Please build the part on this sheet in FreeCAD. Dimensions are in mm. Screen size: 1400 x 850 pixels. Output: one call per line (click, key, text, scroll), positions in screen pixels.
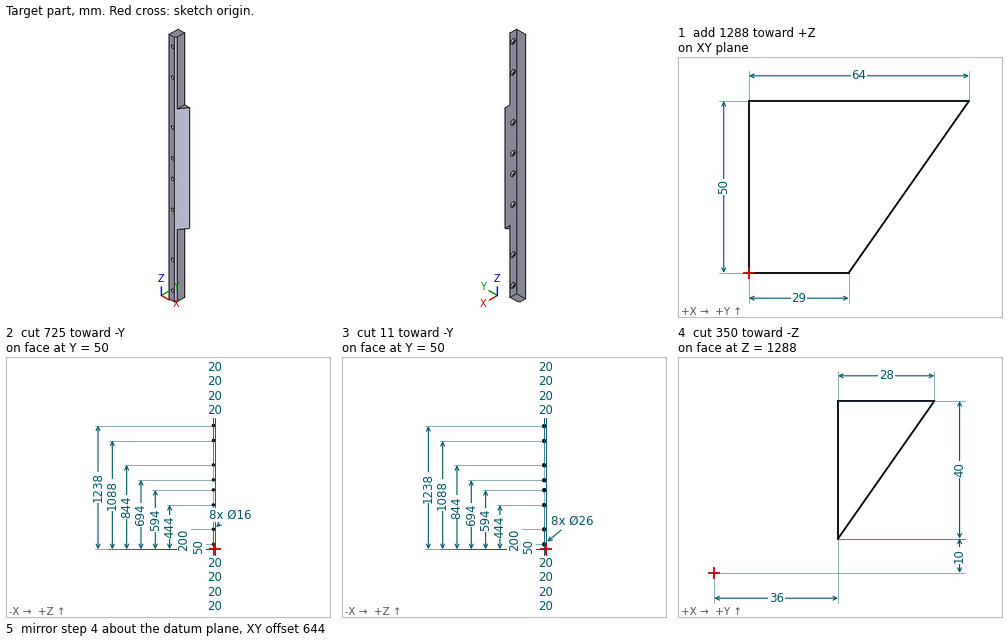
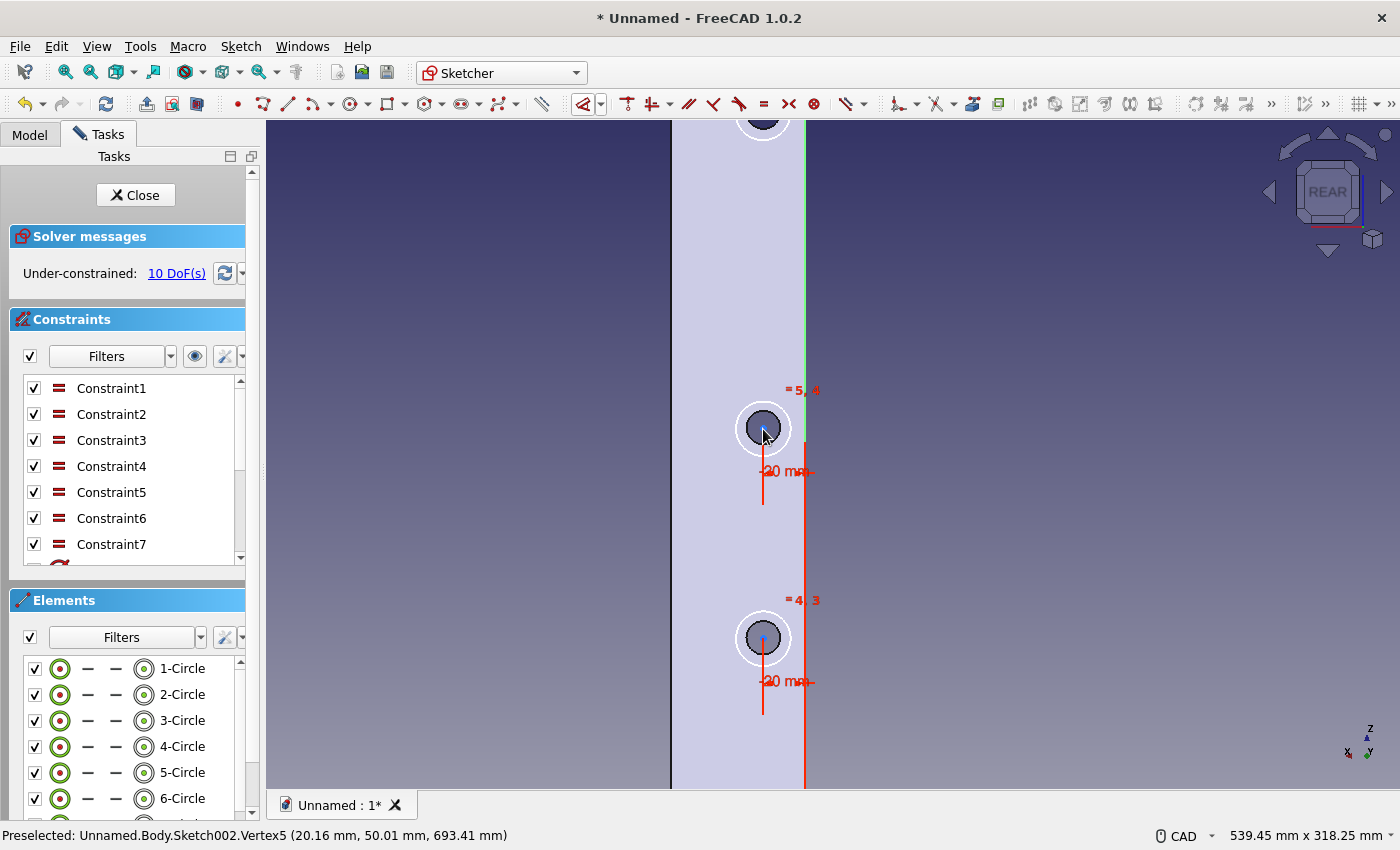
scroll(763, 431, down, 9)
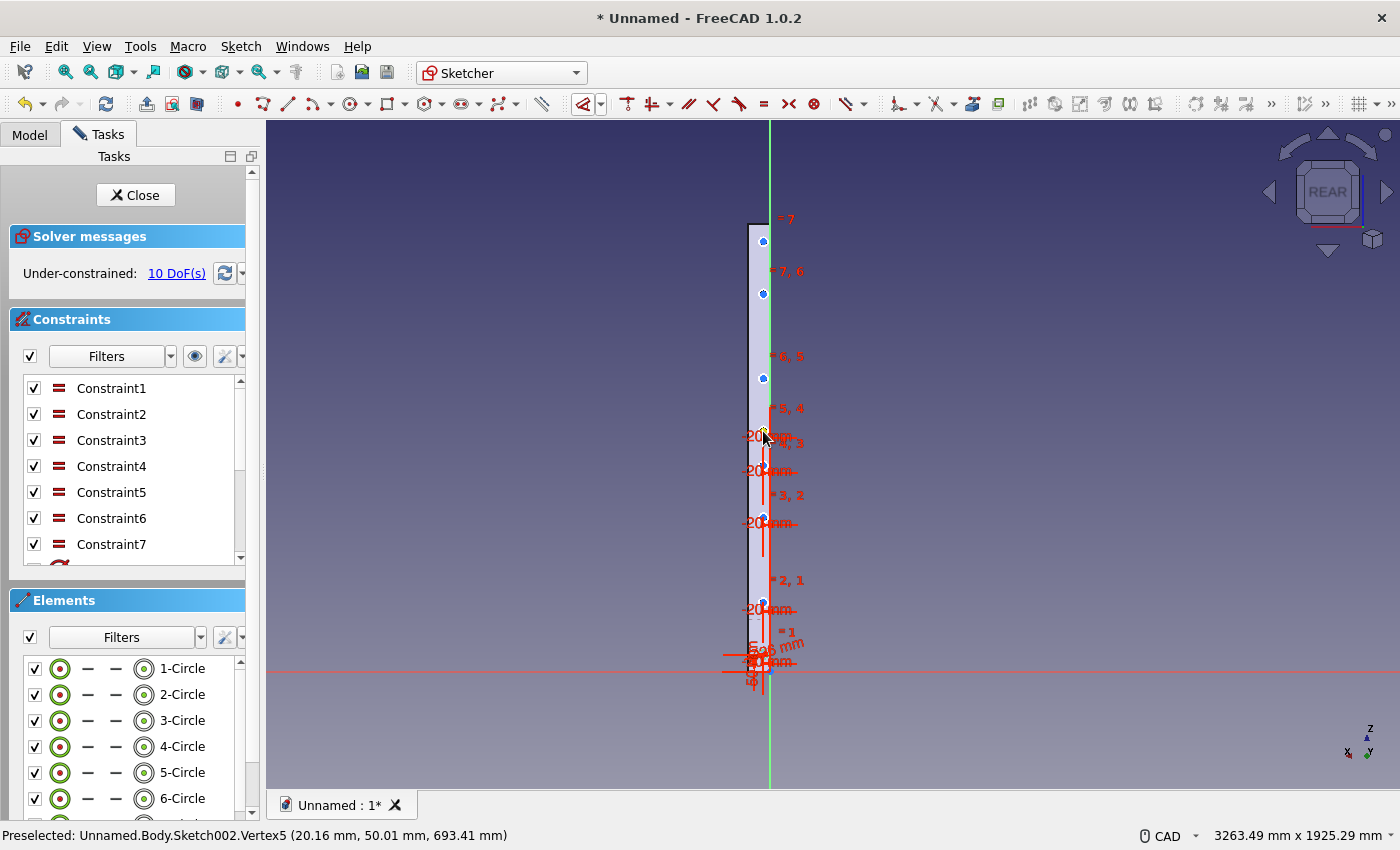
scroll(763, 379, up, 9)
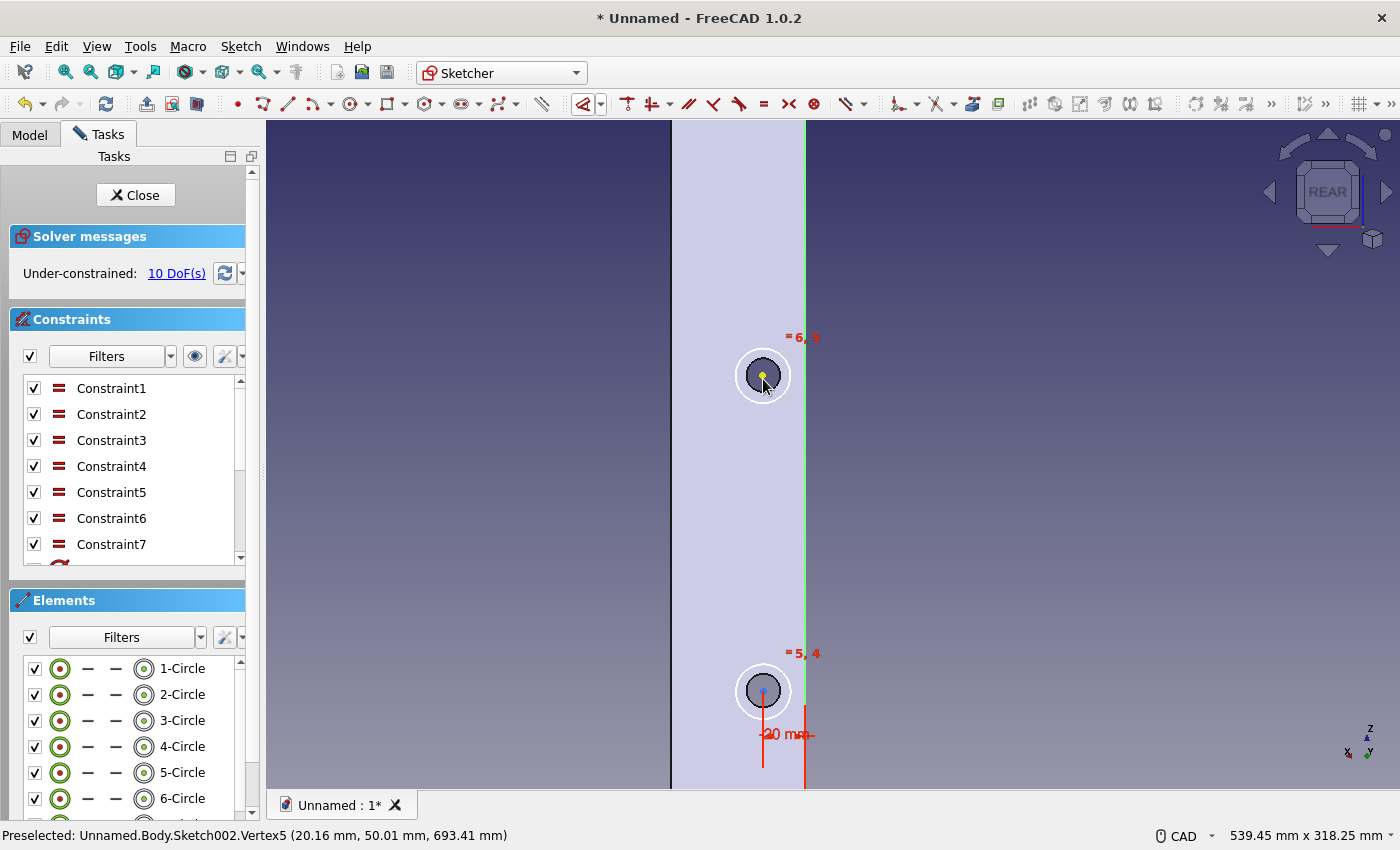
click(763, 376)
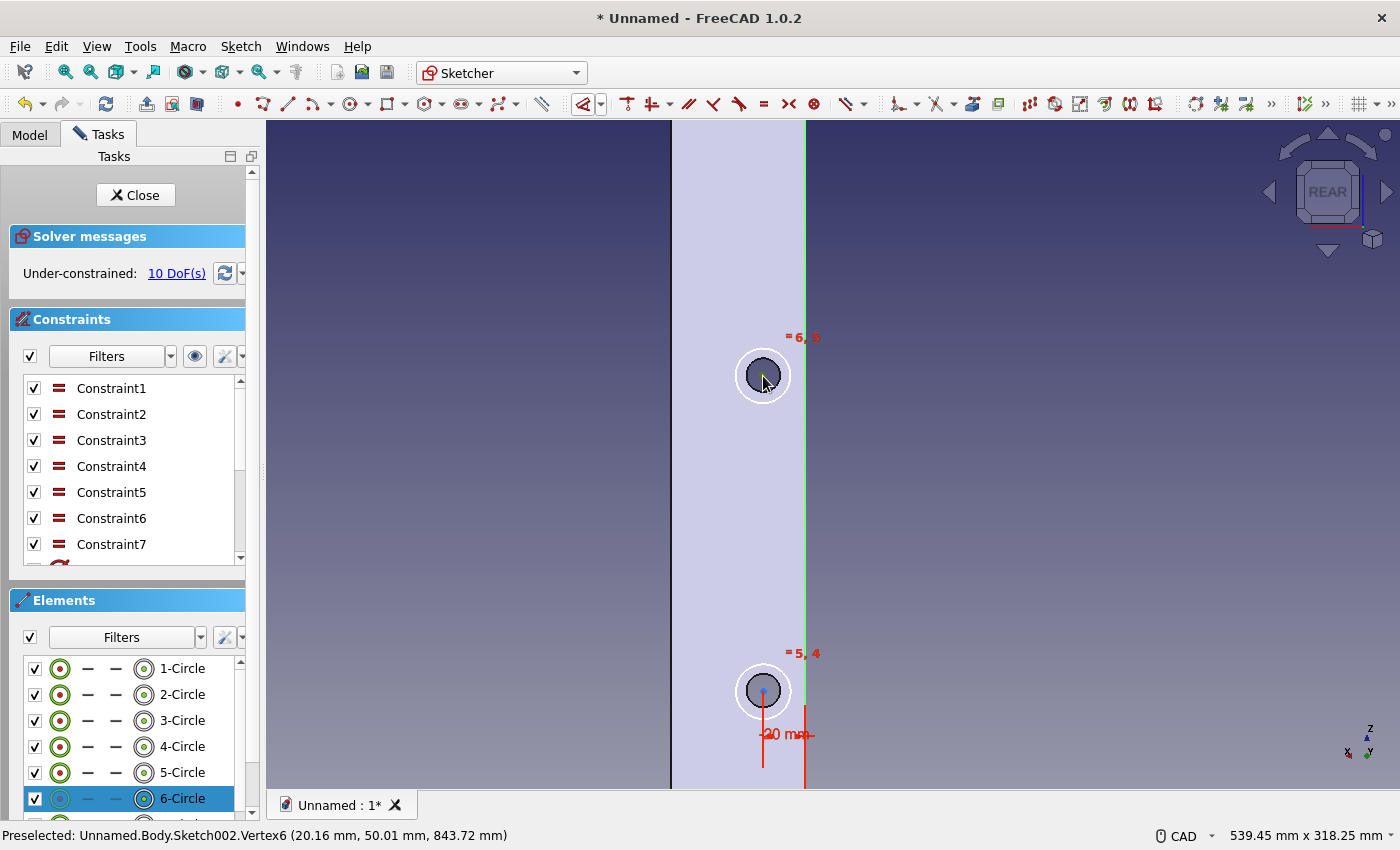
key(l)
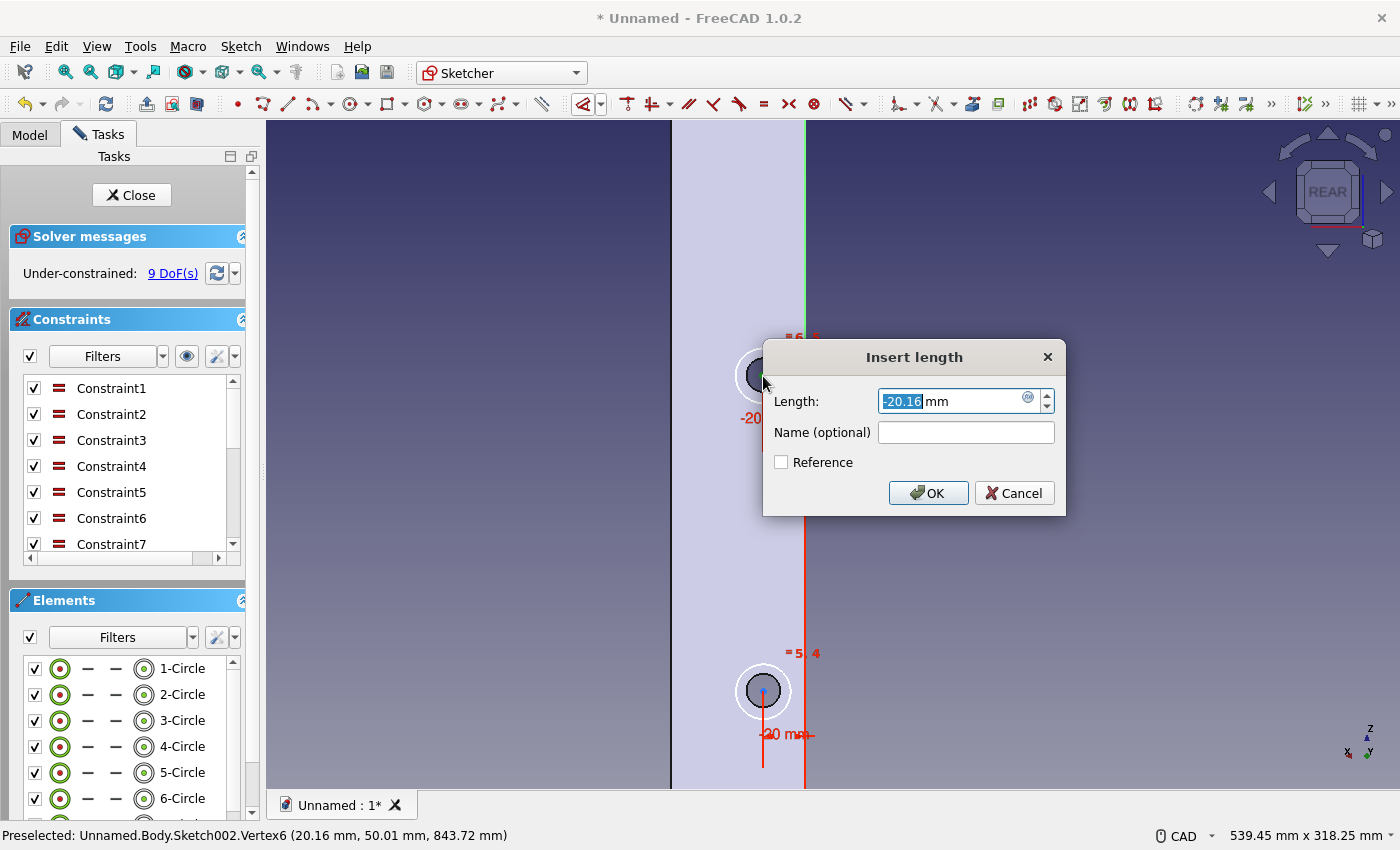
text(-20)
key(Return)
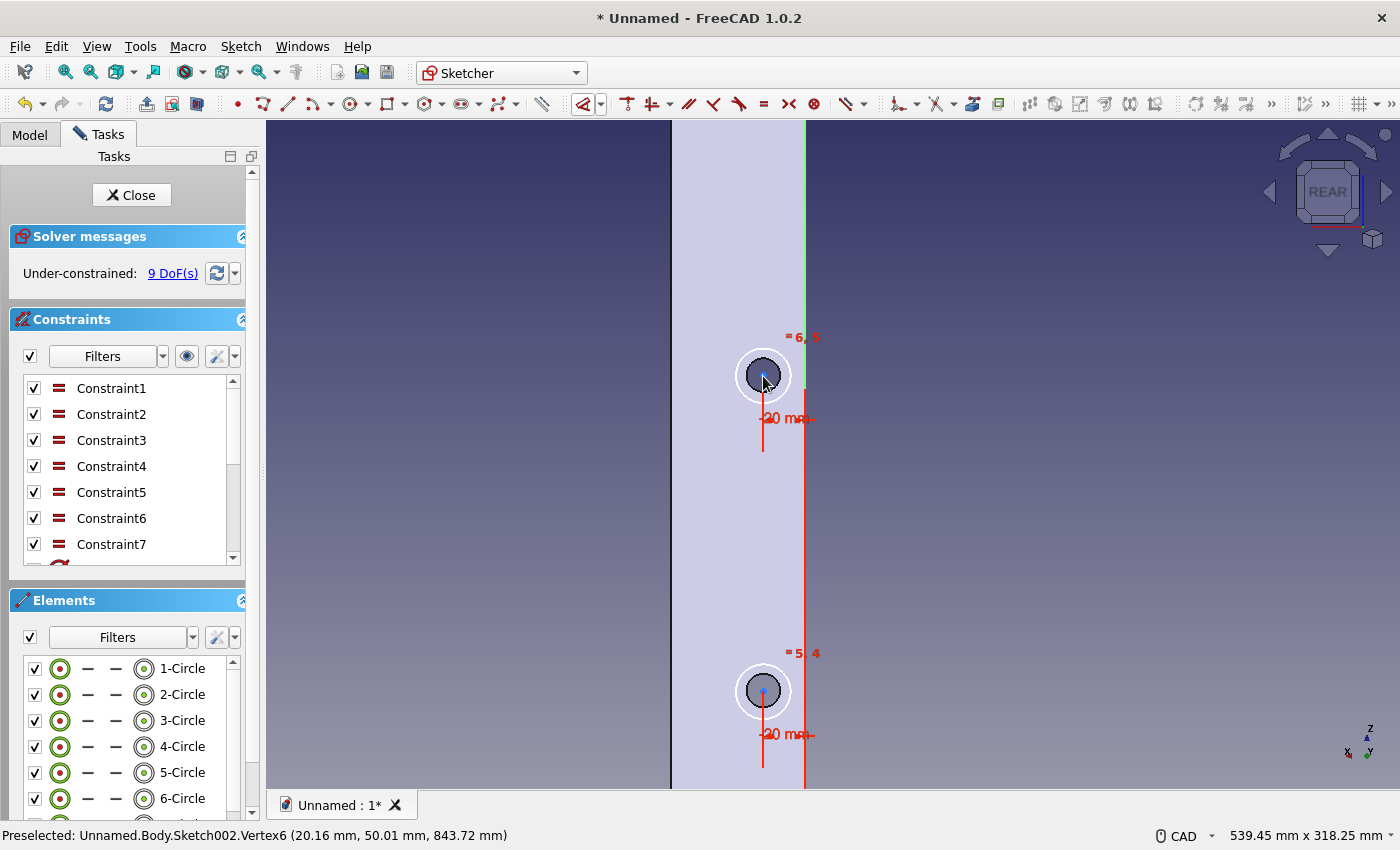
scroll(763, 379, down, 9)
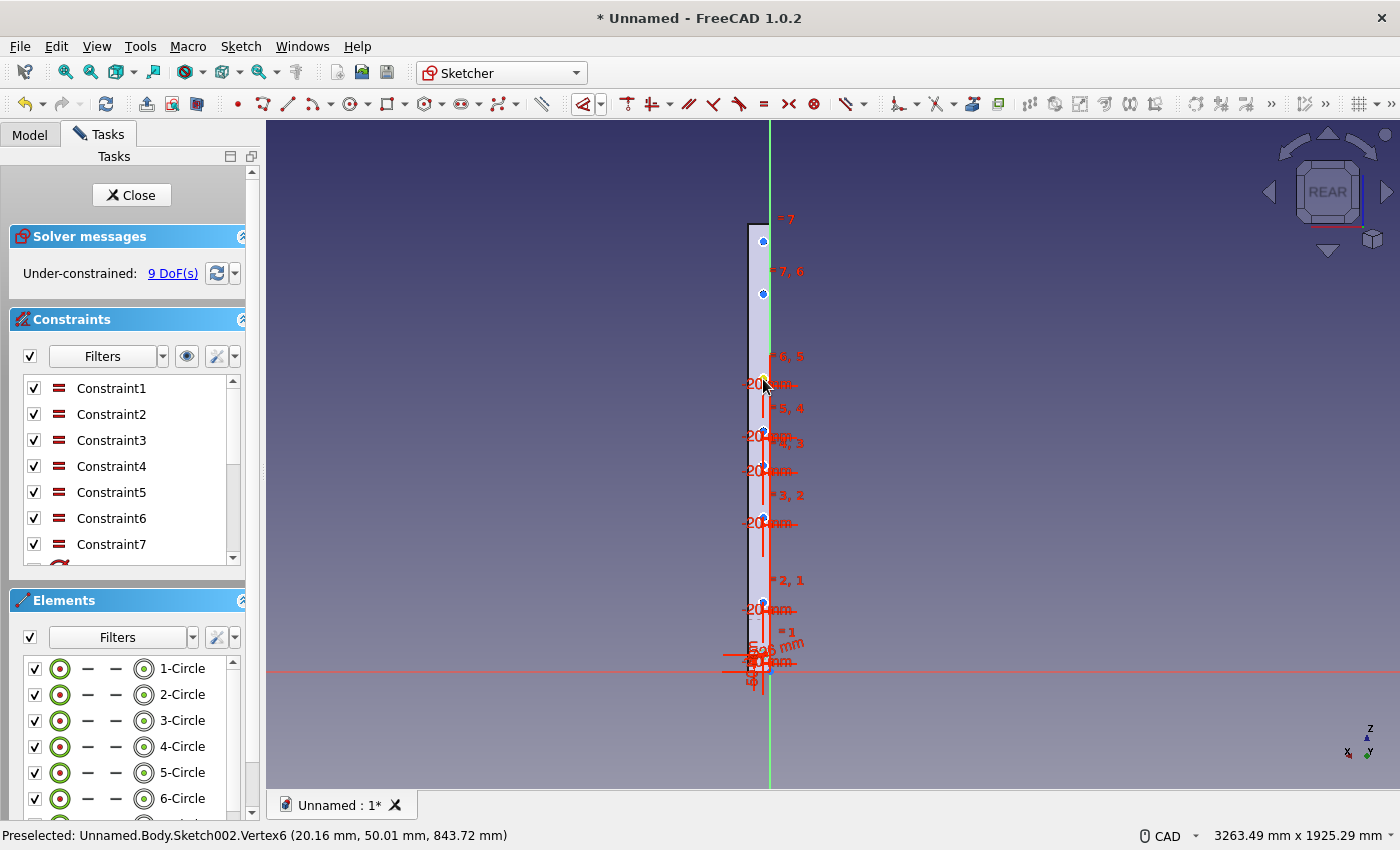
scroll(763, 294, up, 9)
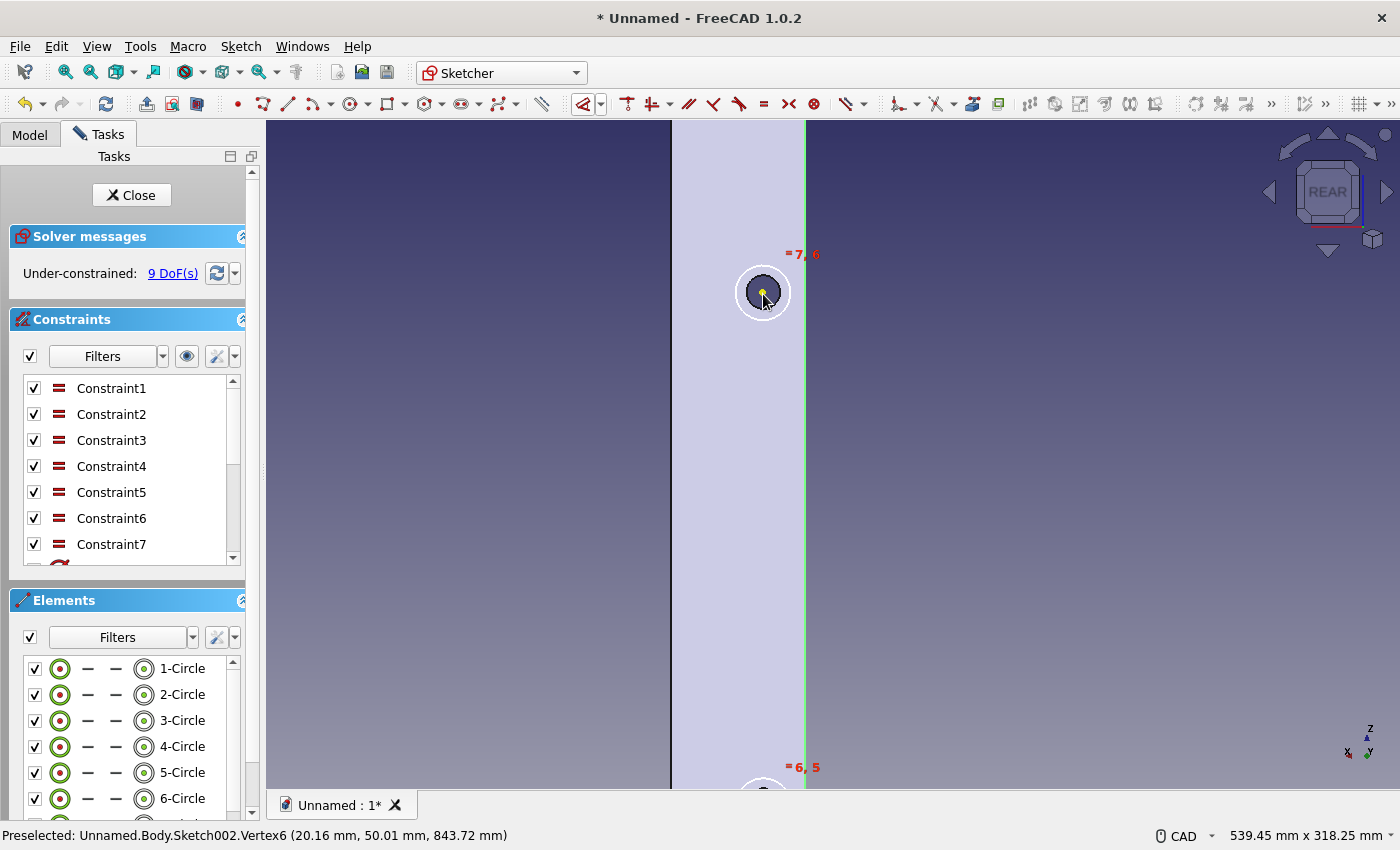
click(763, 293)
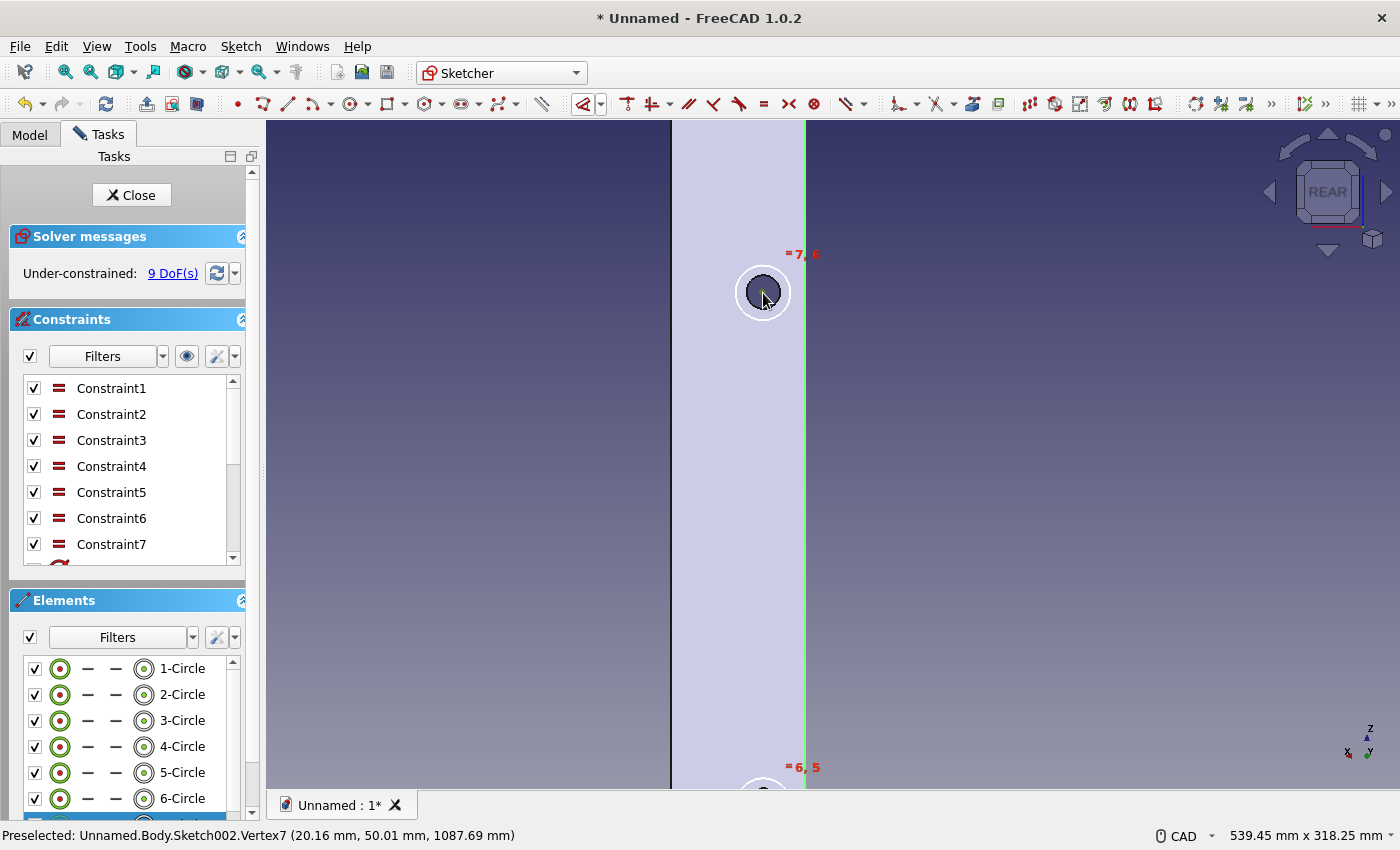
key(l)